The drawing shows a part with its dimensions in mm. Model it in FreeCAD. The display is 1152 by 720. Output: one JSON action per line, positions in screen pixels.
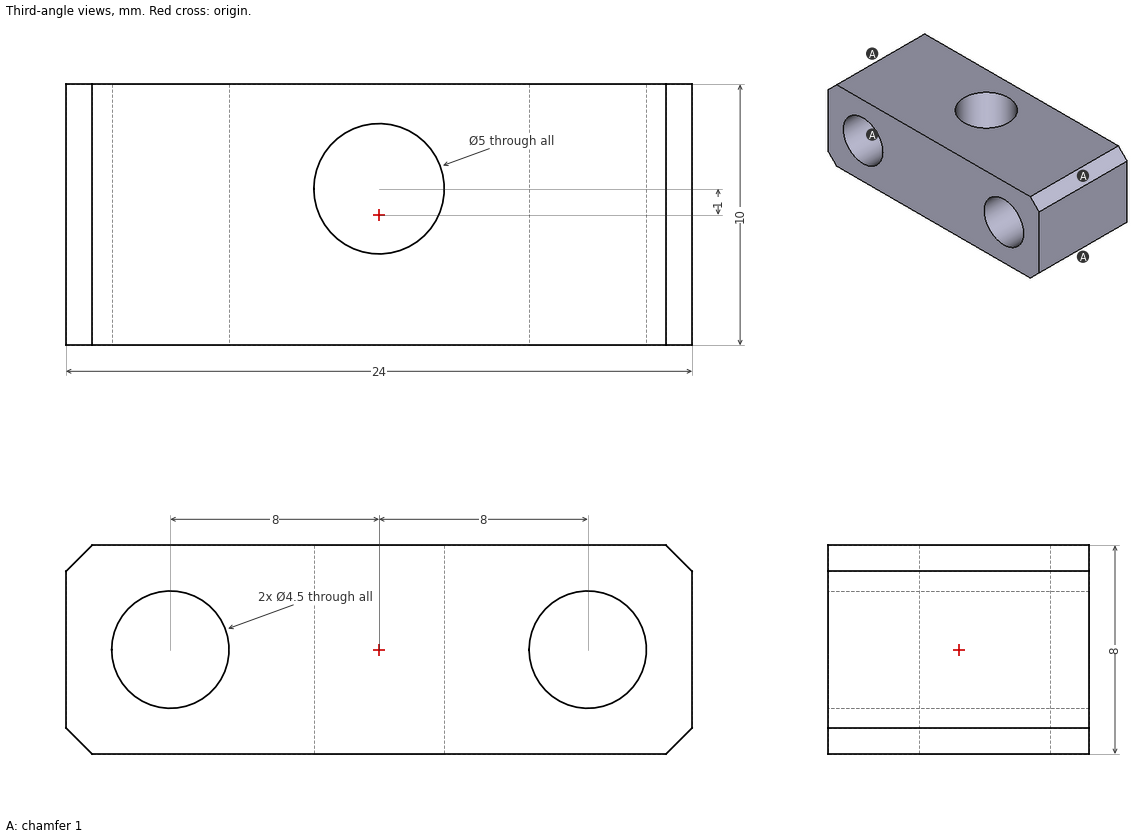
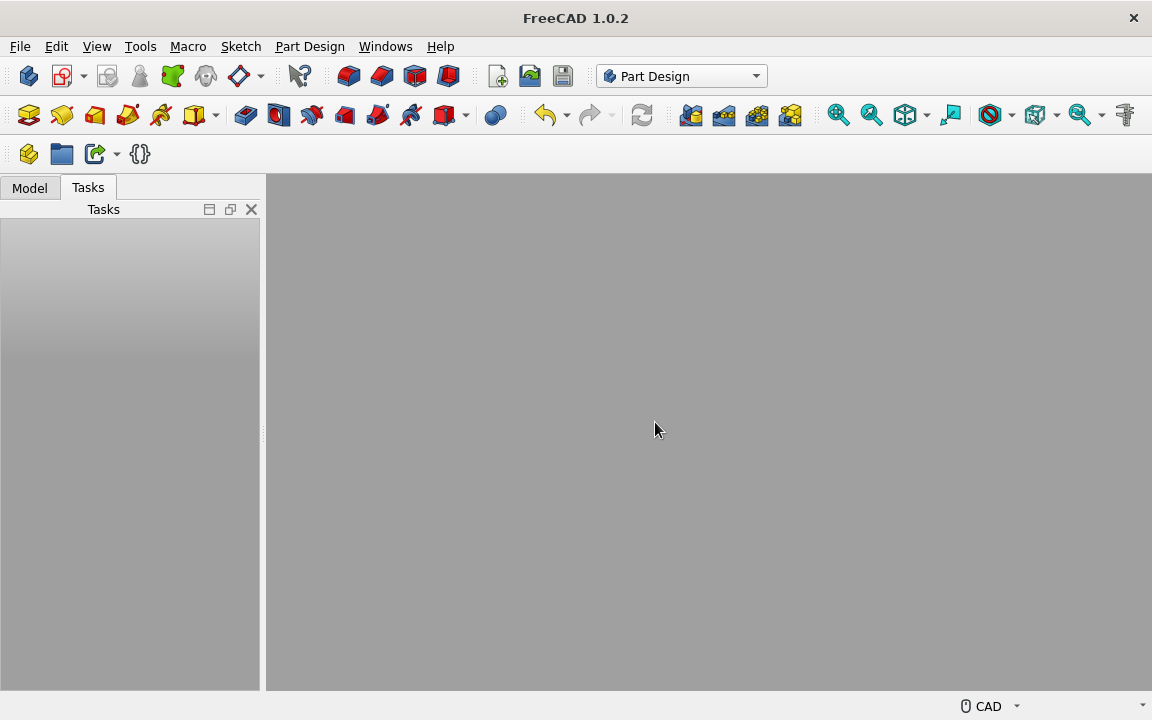
{"action": "left_click", "coordinate": [497, 76]}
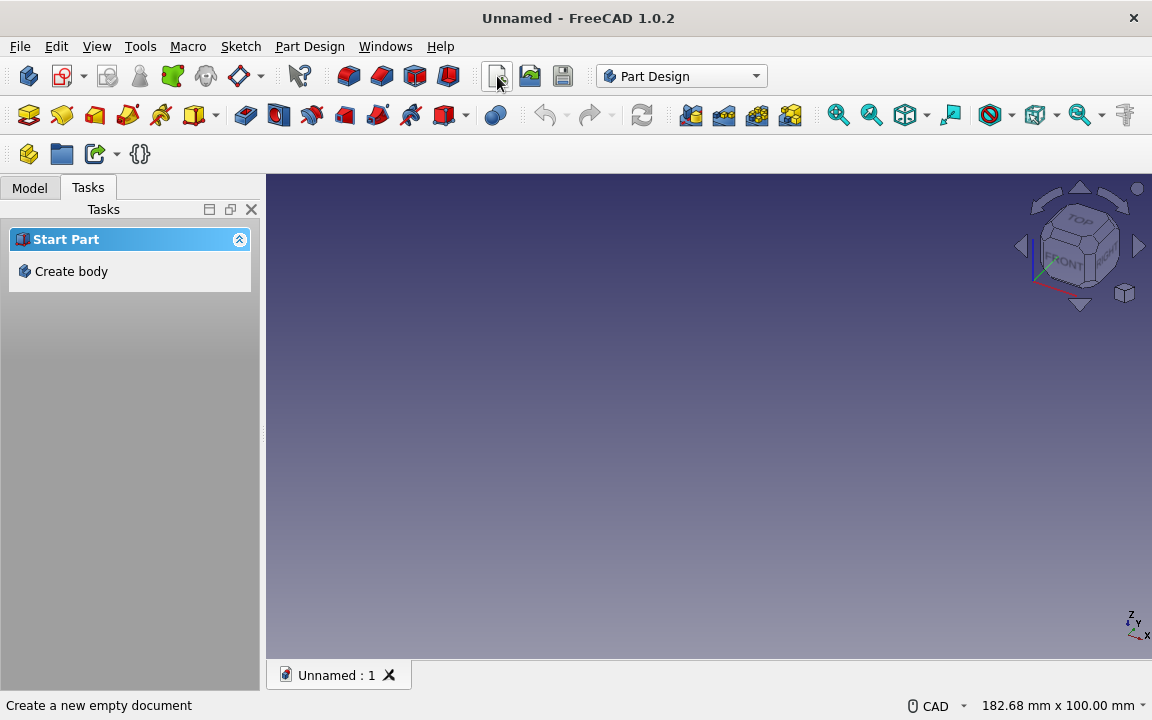
{"action": "left_click", "coordinate": [62, 76]}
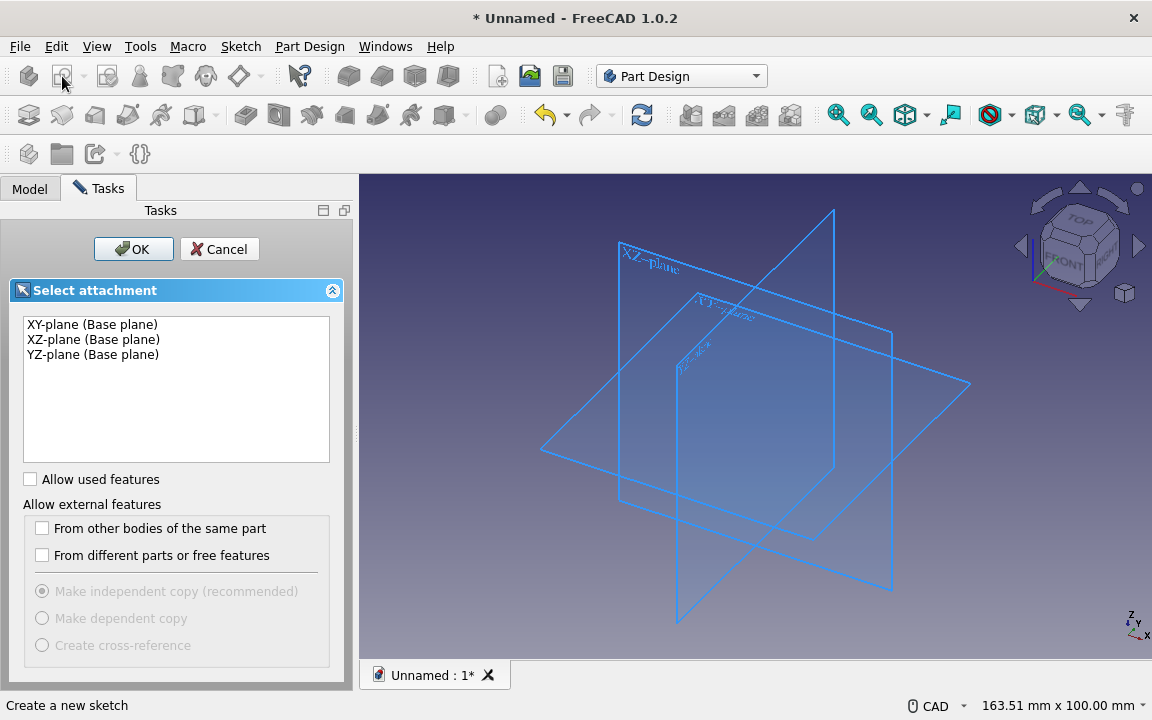
{"action": "left_click", "coordinate": [84, 324]}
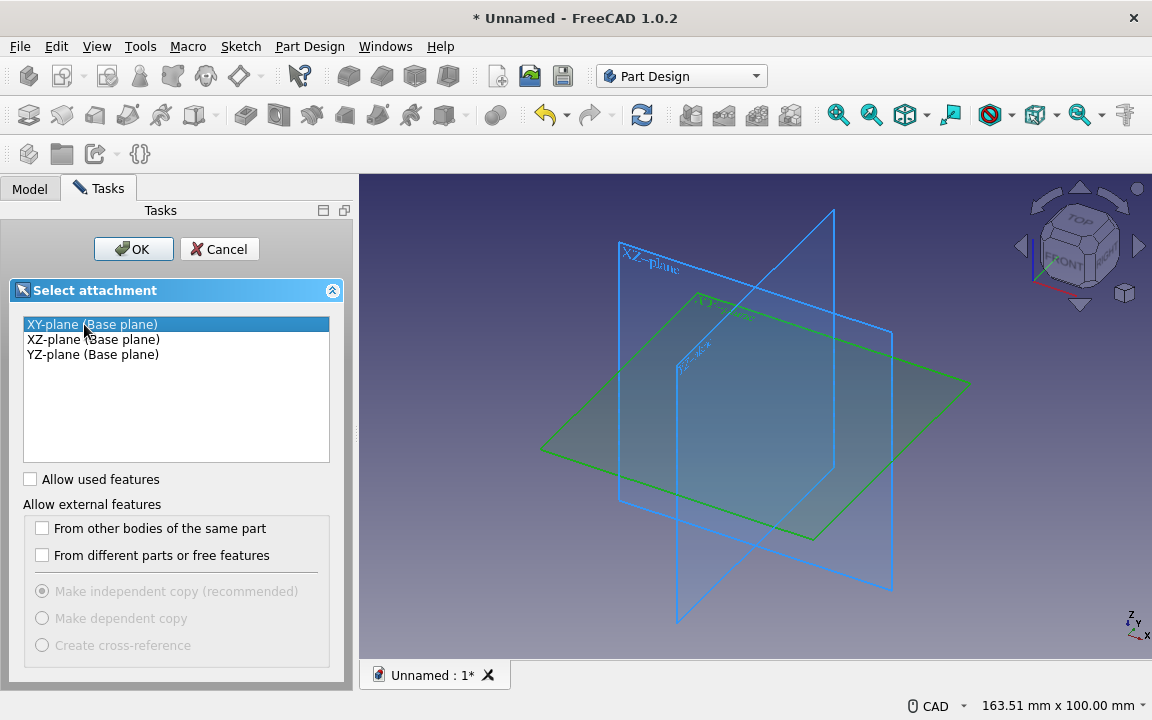
{"action": "left_click", "coordinate": [134, 249]}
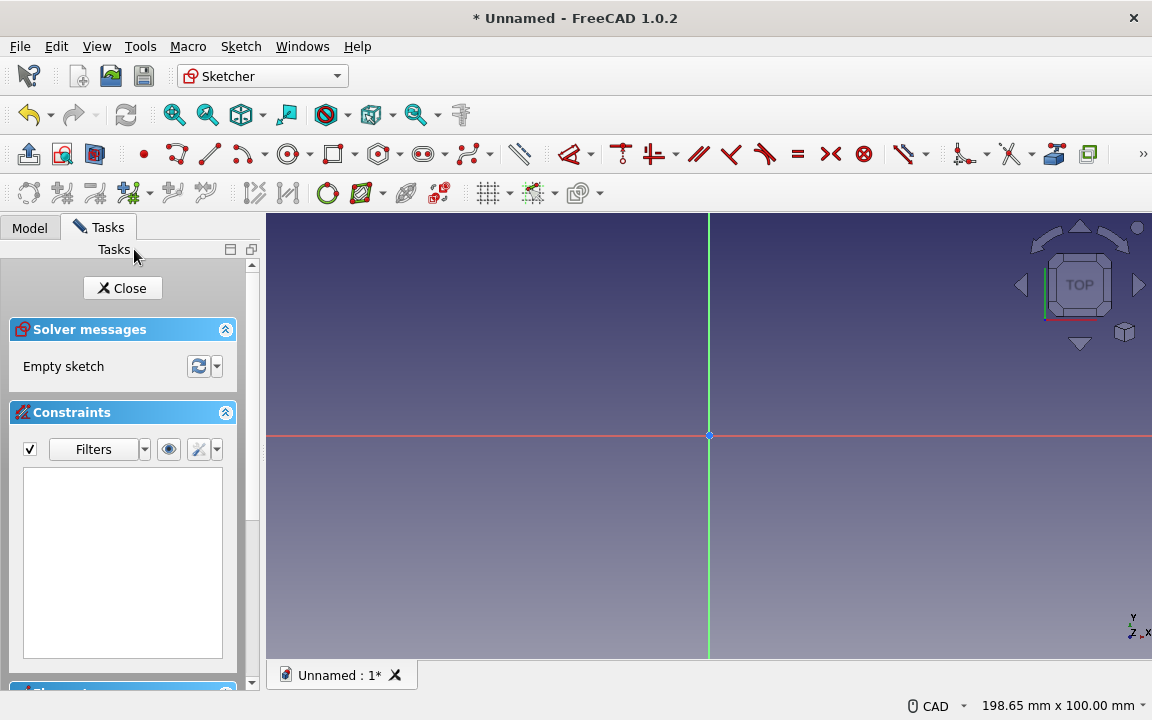
{"action": "scroll", "coordinate": [726, 436], "scroll_direction": "up", "scroll_amount": 8}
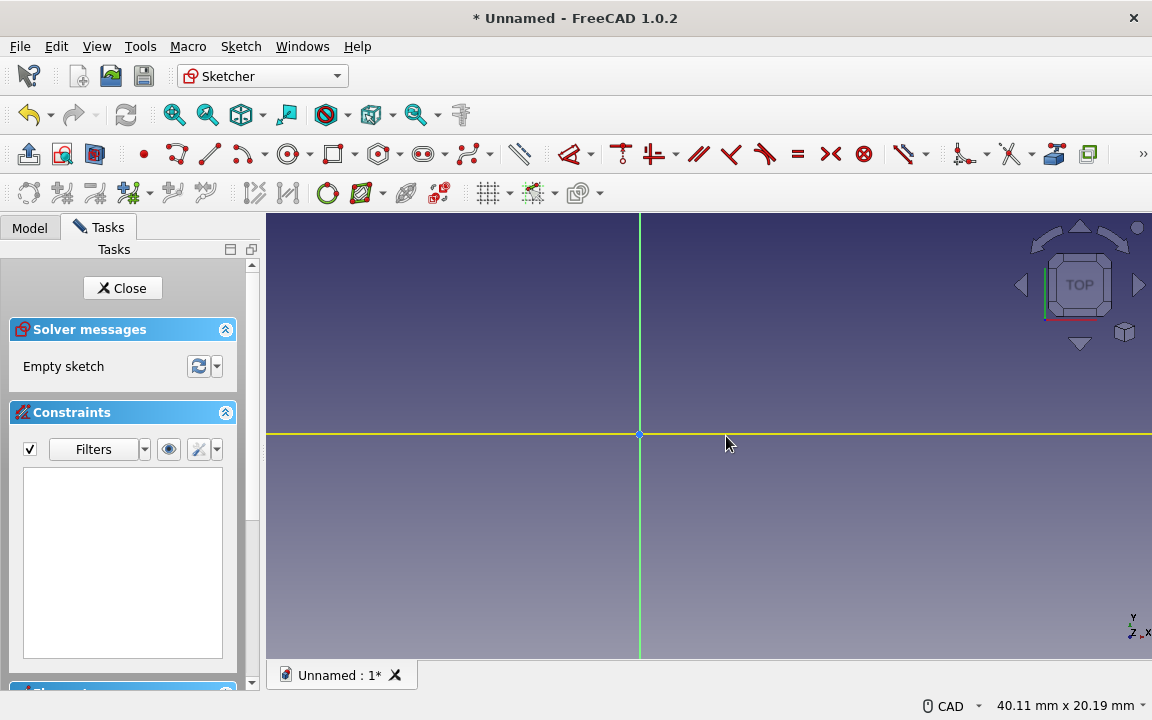
{"action": "key", "text": "g v"}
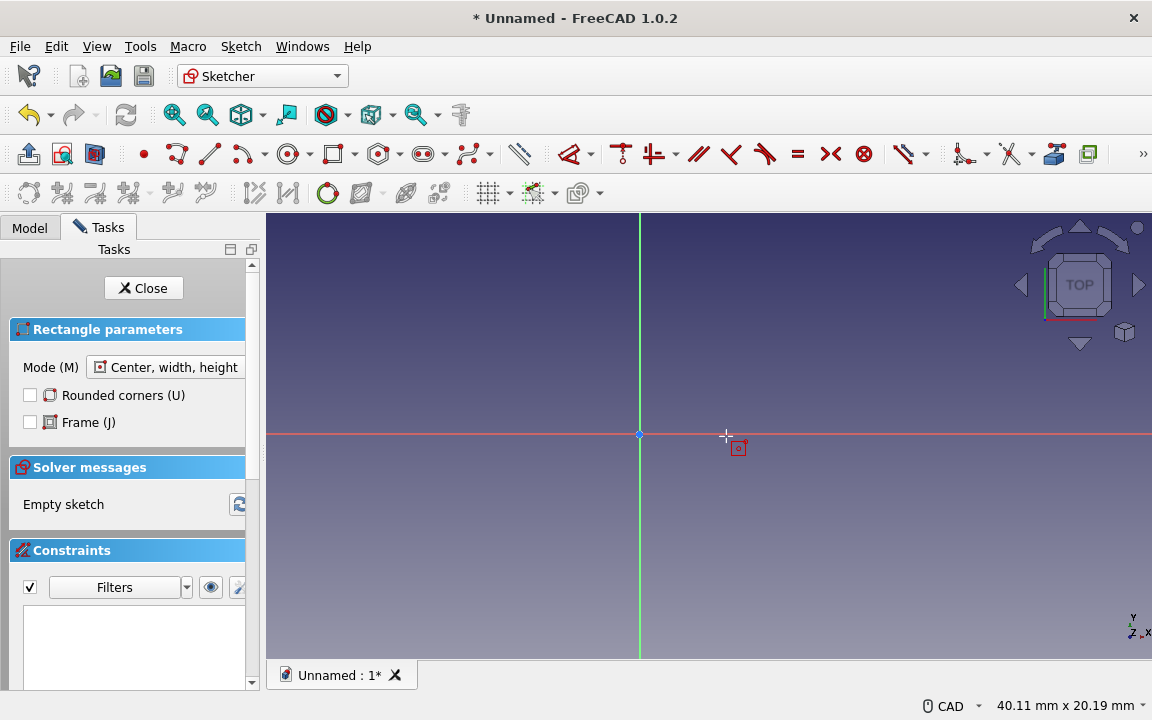
{"action": "left_click", "coordinate": [640, 434]}
{"action": "left_click", "coordinate": [905, 324]}
{"action": "key", "text": "Escape"}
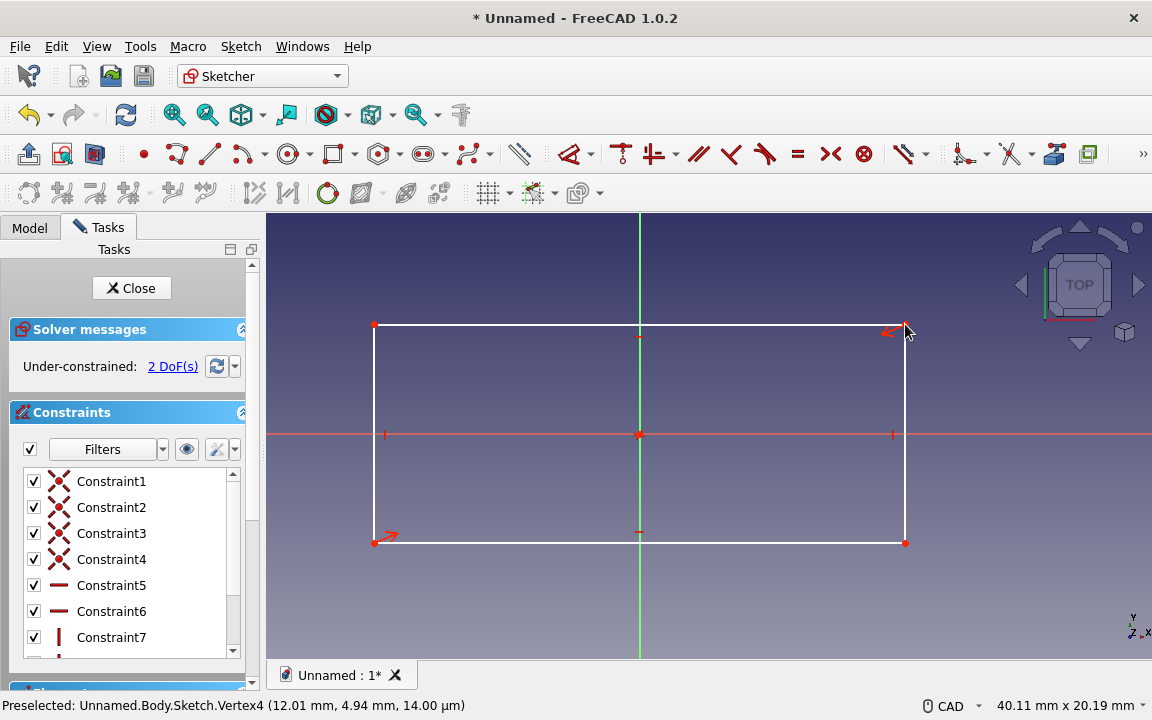
{"action": "left_click", "coordinate": [534, 543]}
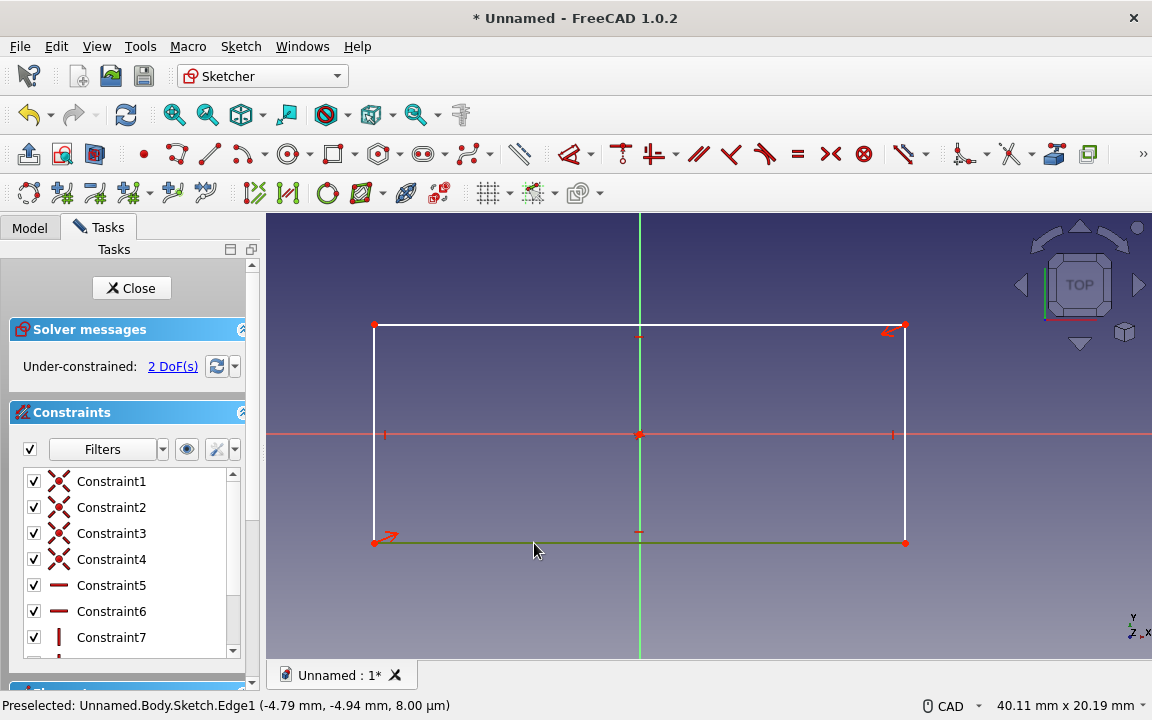
{"action": "key", "text": "l"}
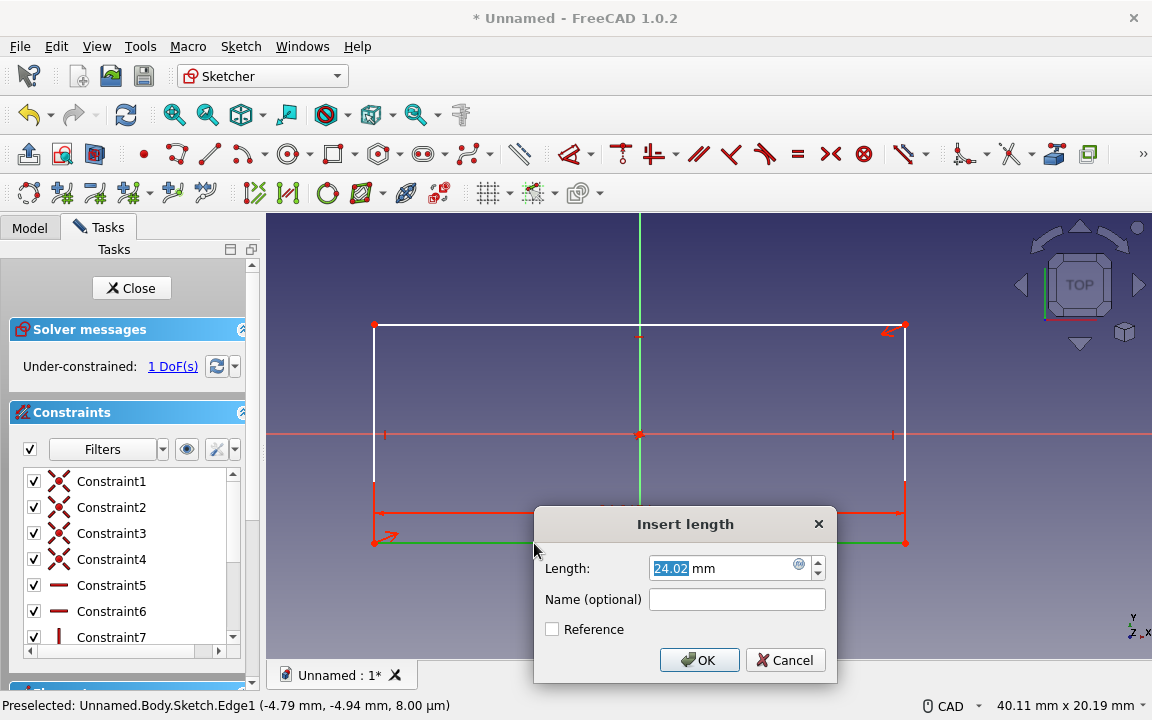
{"action": "type", "text": "24"}
{"action": "key", "text": "Return"}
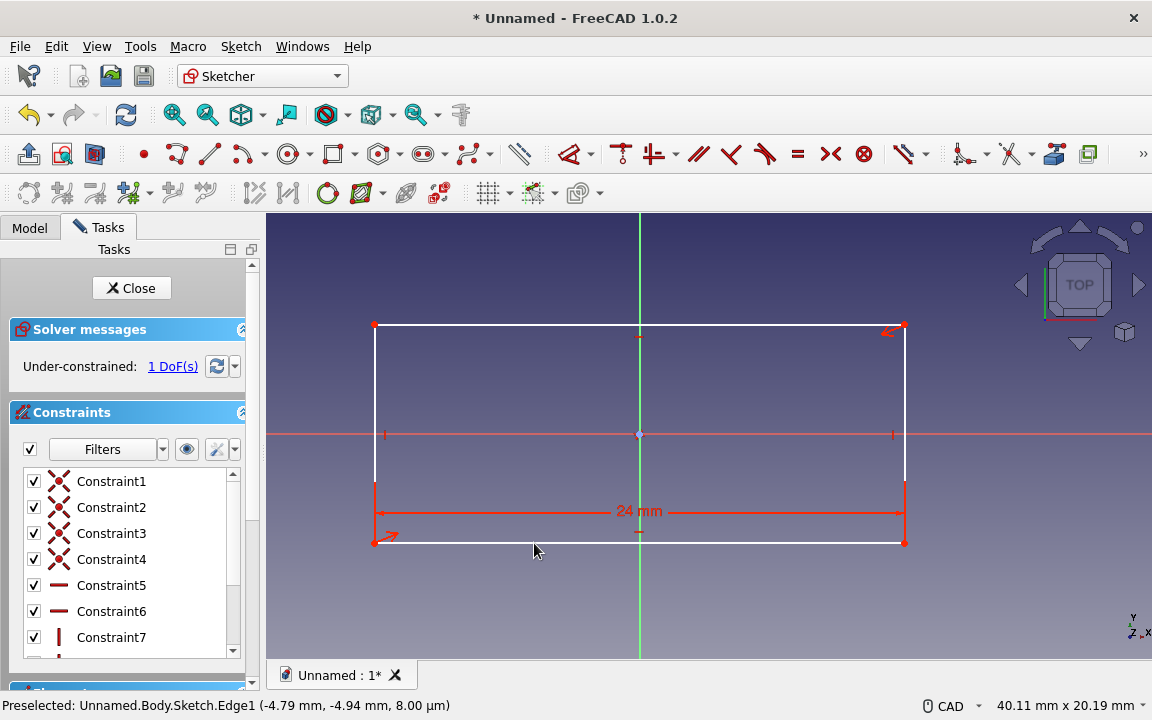
{"action": "left_click", "coordinate": [905, 478]}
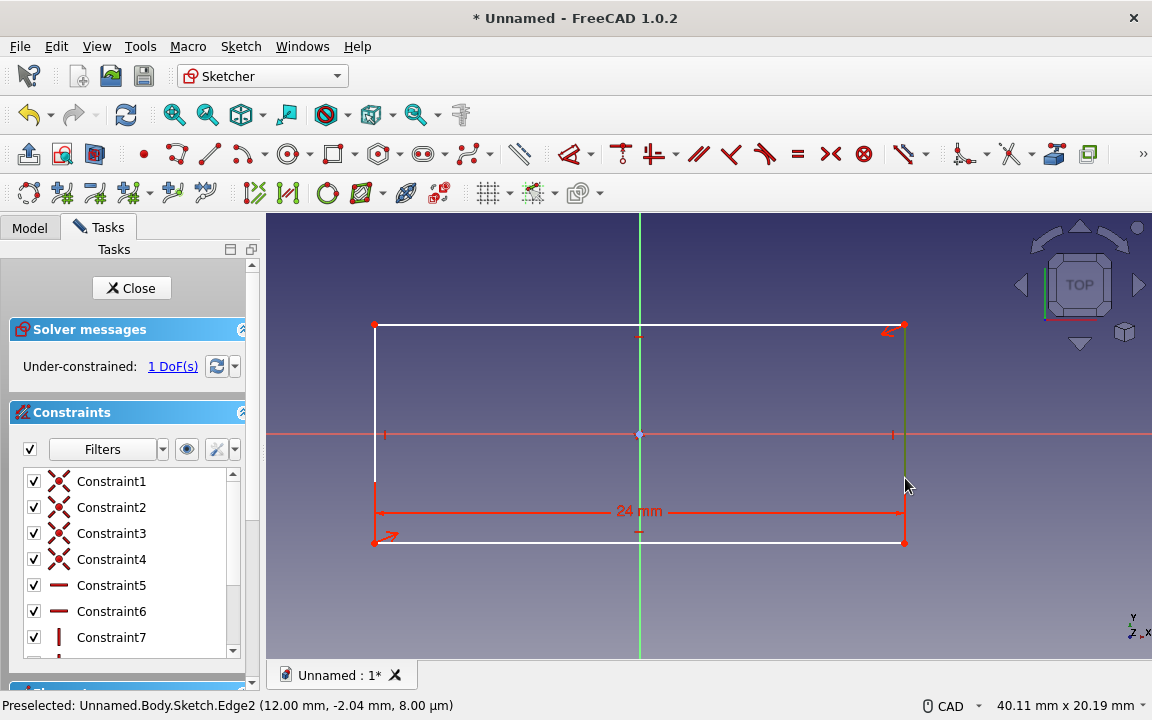
{"action": "left_click", "coordinate": [590, 154]}